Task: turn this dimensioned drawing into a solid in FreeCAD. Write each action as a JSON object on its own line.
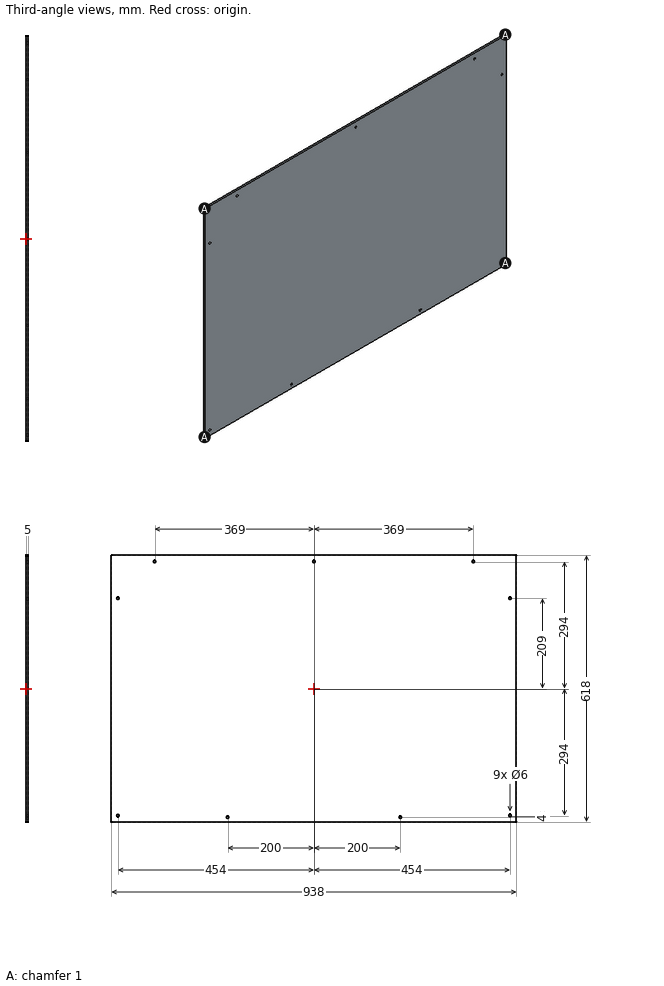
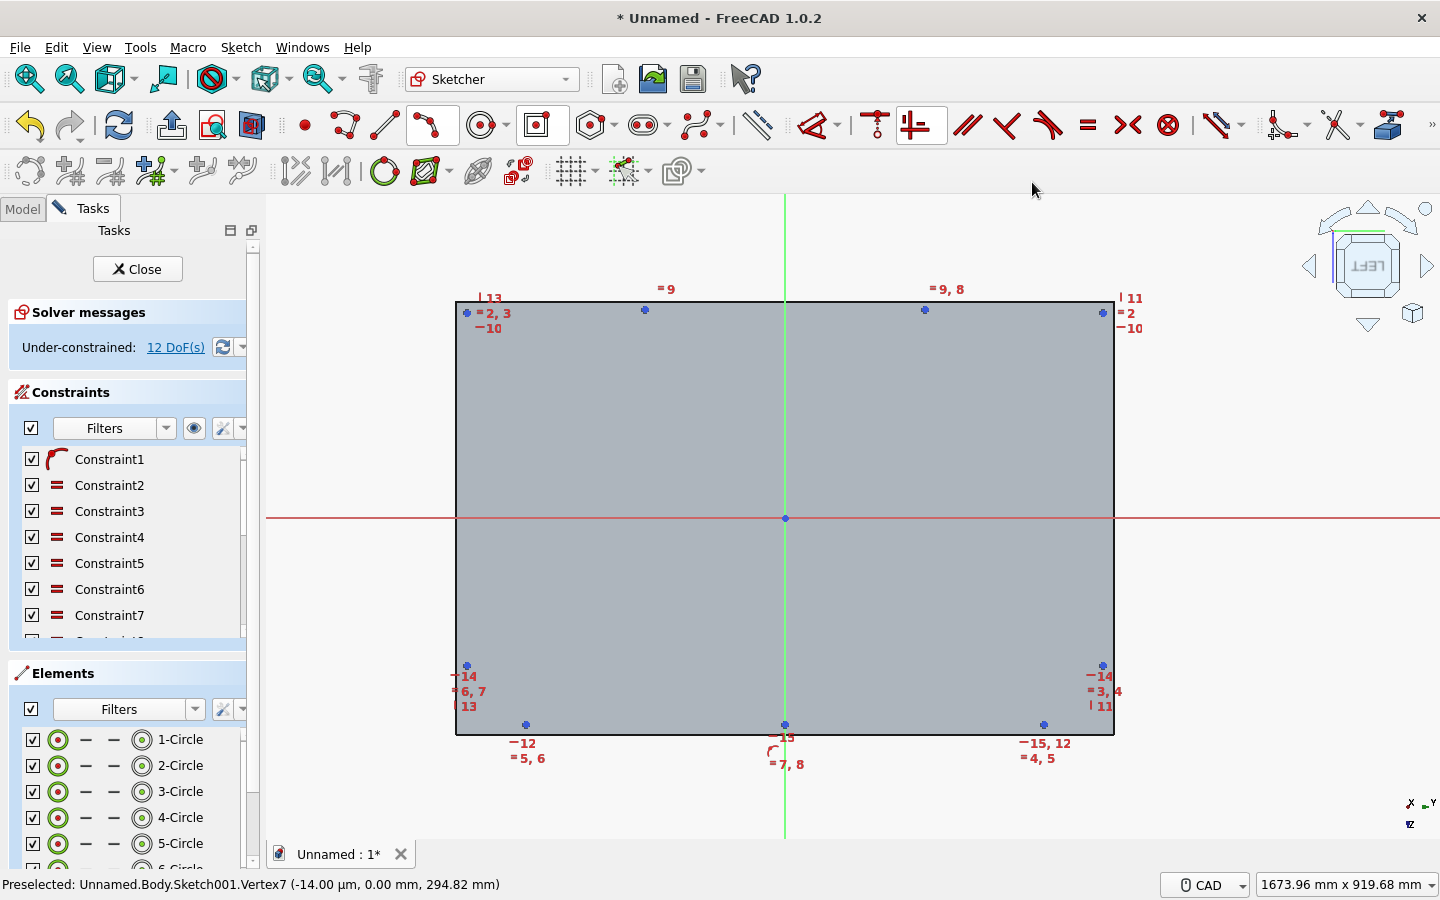
{"action": "left_click", "coordinate": [925, 310]}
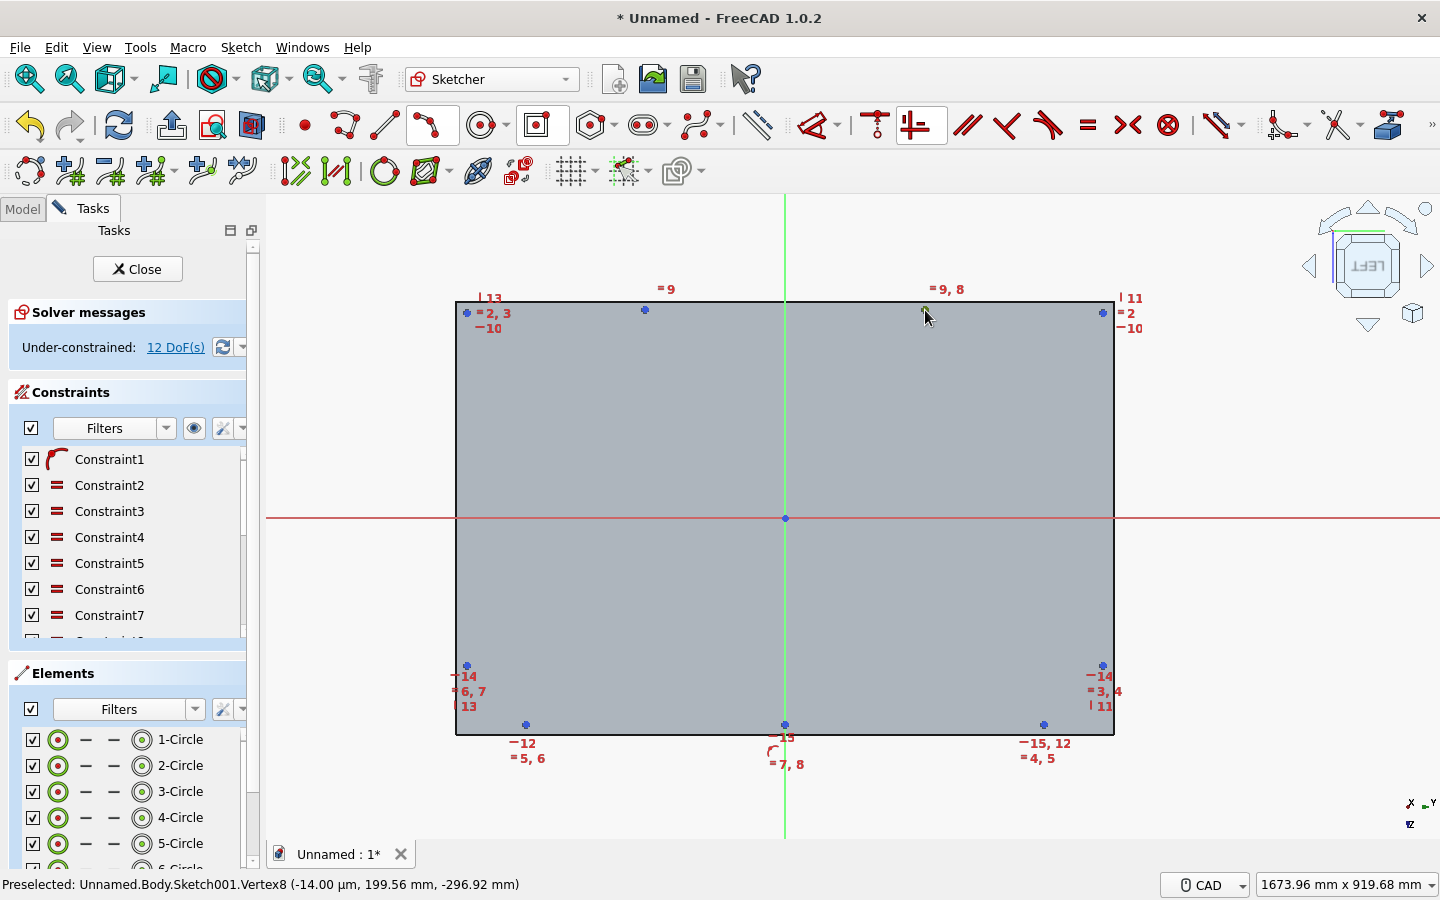
{"action": "left_click", "coordinate": [645, 310]}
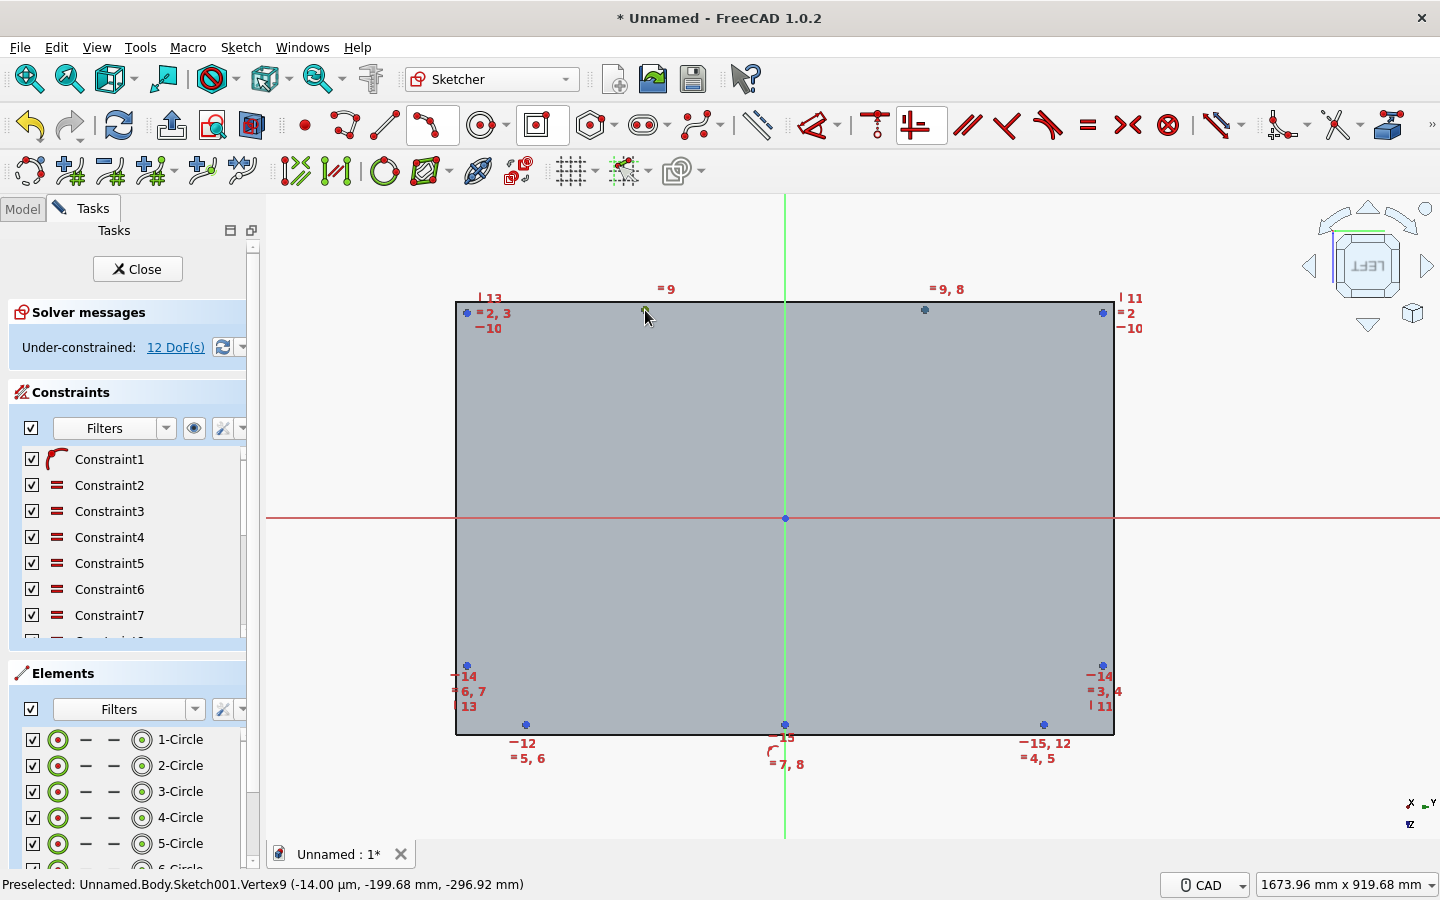
{"action": "key", "text": "h"}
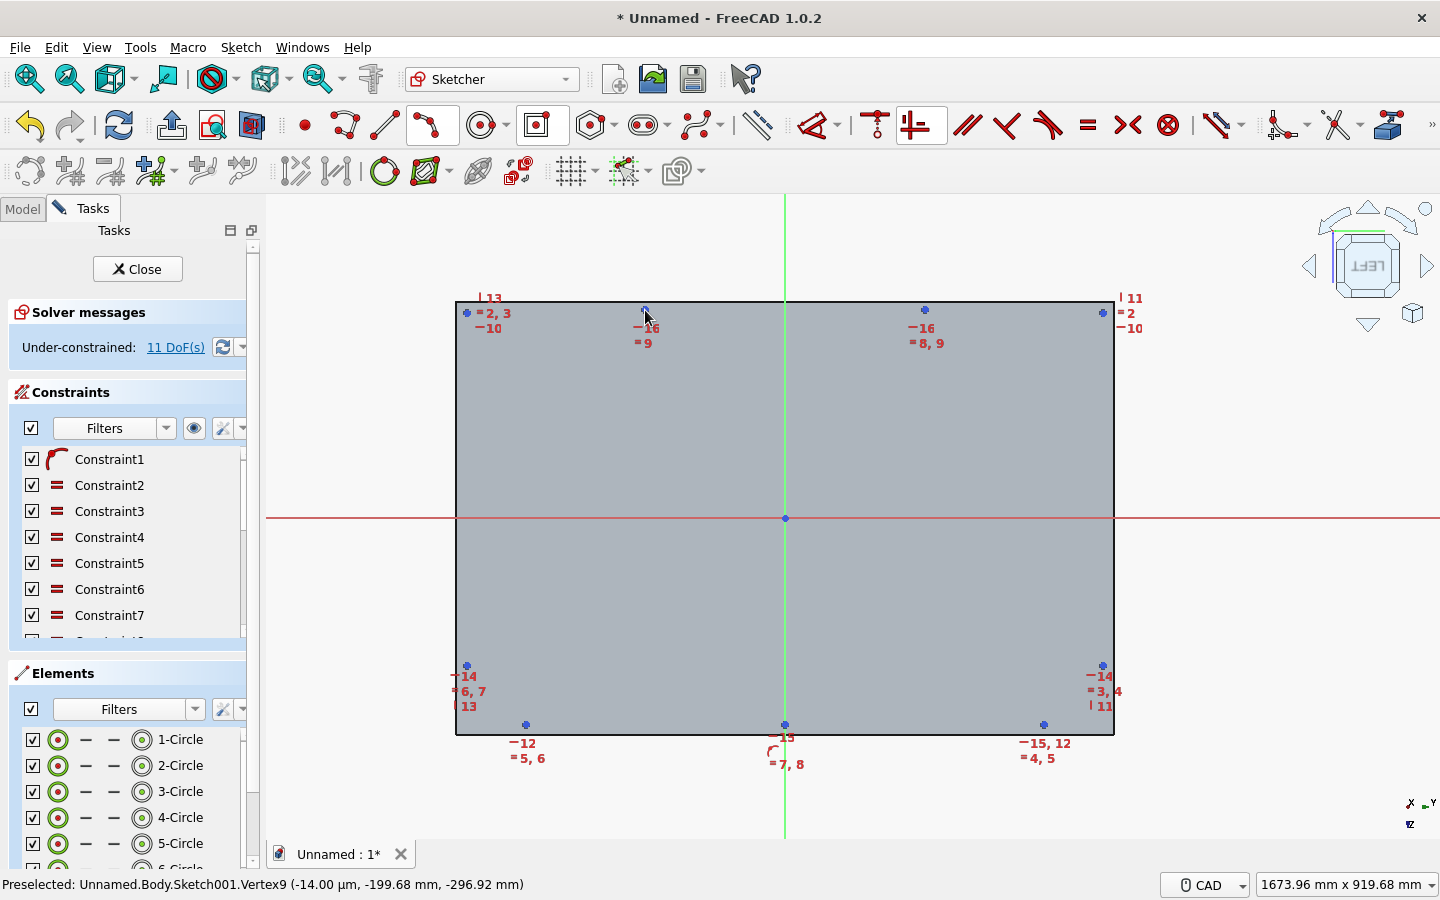
{"action": "left_click", "coordinate": [812, 126]}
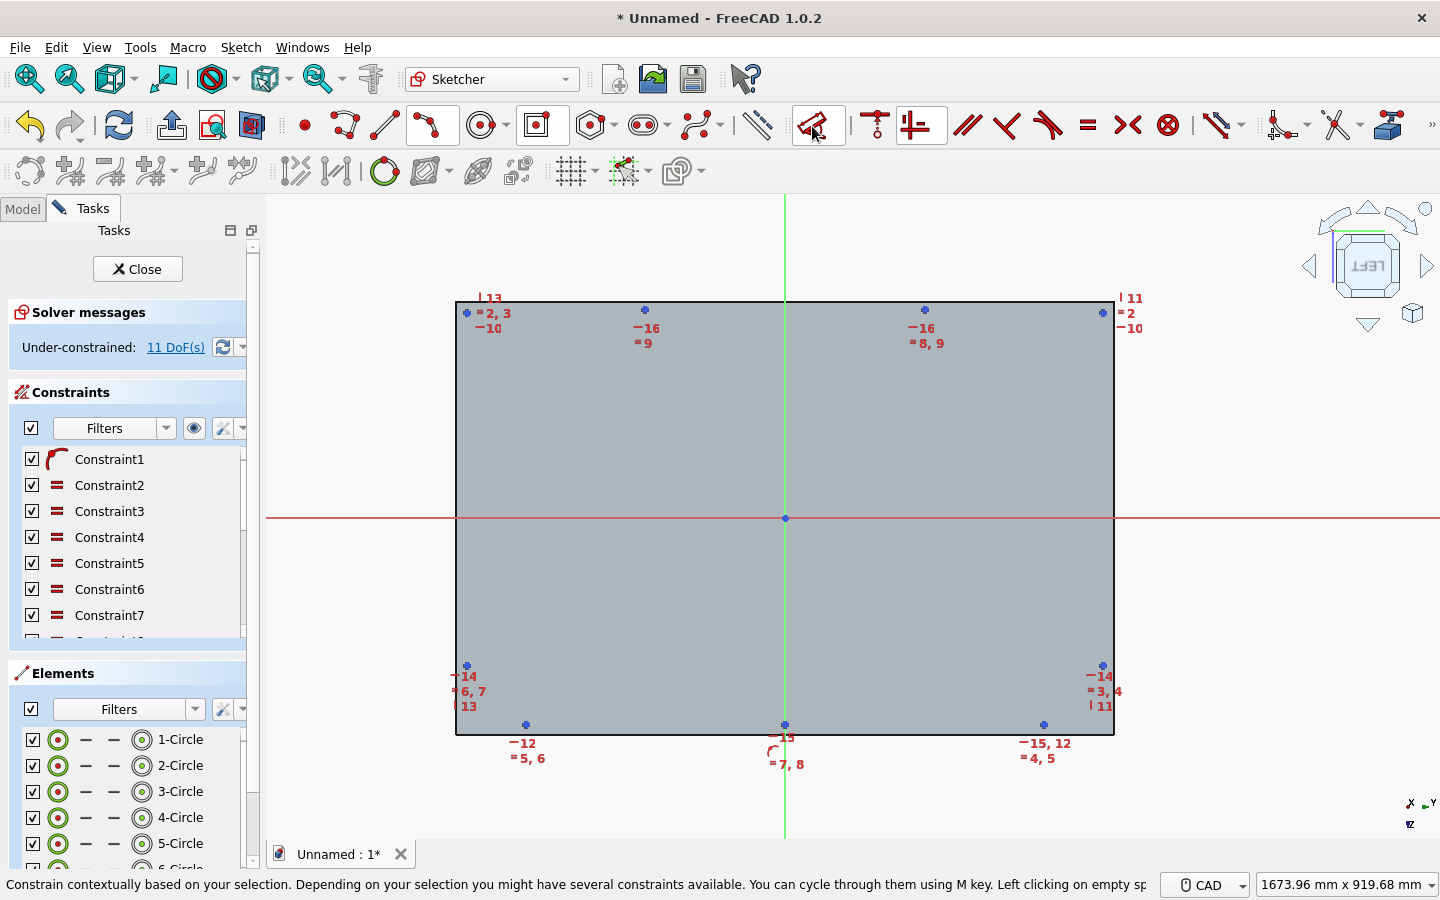
{"action": "scroll", "coordinate": [1105, 311], "scroll_direction": "up", "scroll_amount": 12}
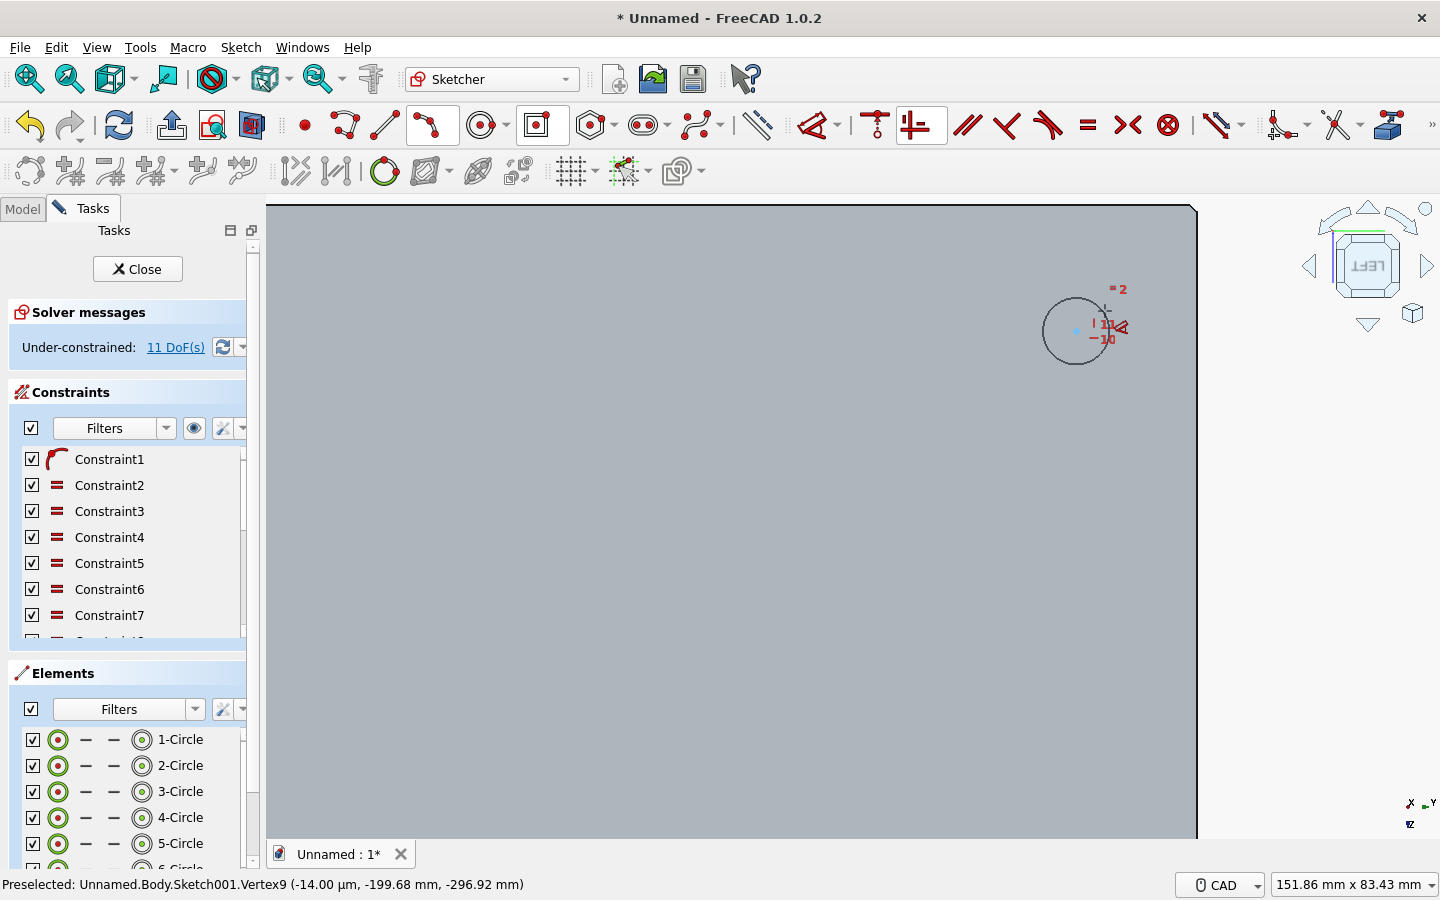
{"action": "left_click", "coordinate": [1100, 308]}
{"action": "left_click", "coordinate": [1123, 286]}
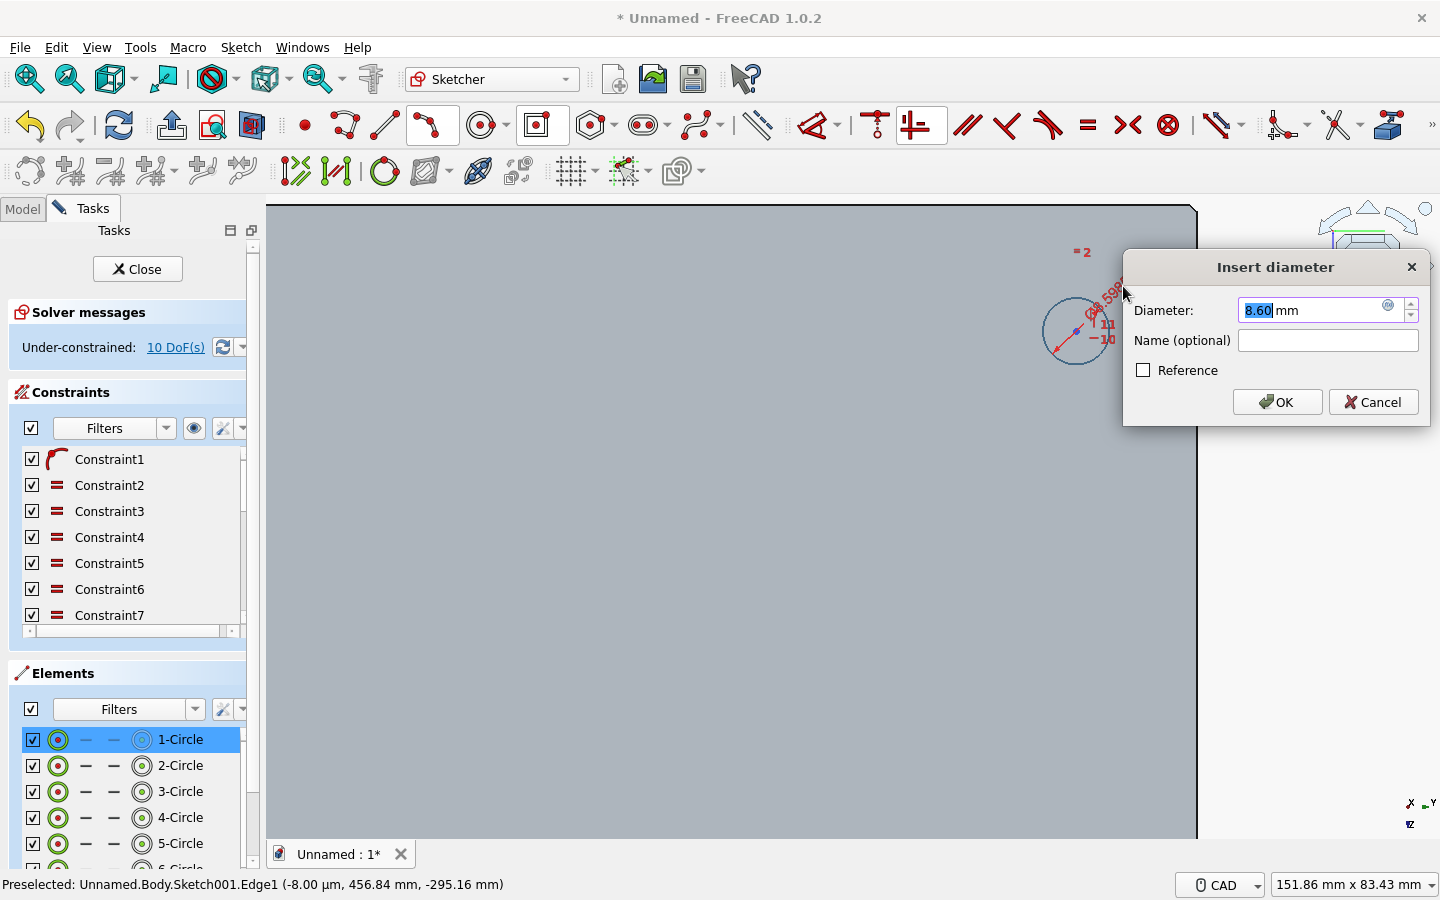
{"action": "type", "text": "6"}
{"action": "key", "text": "Return"}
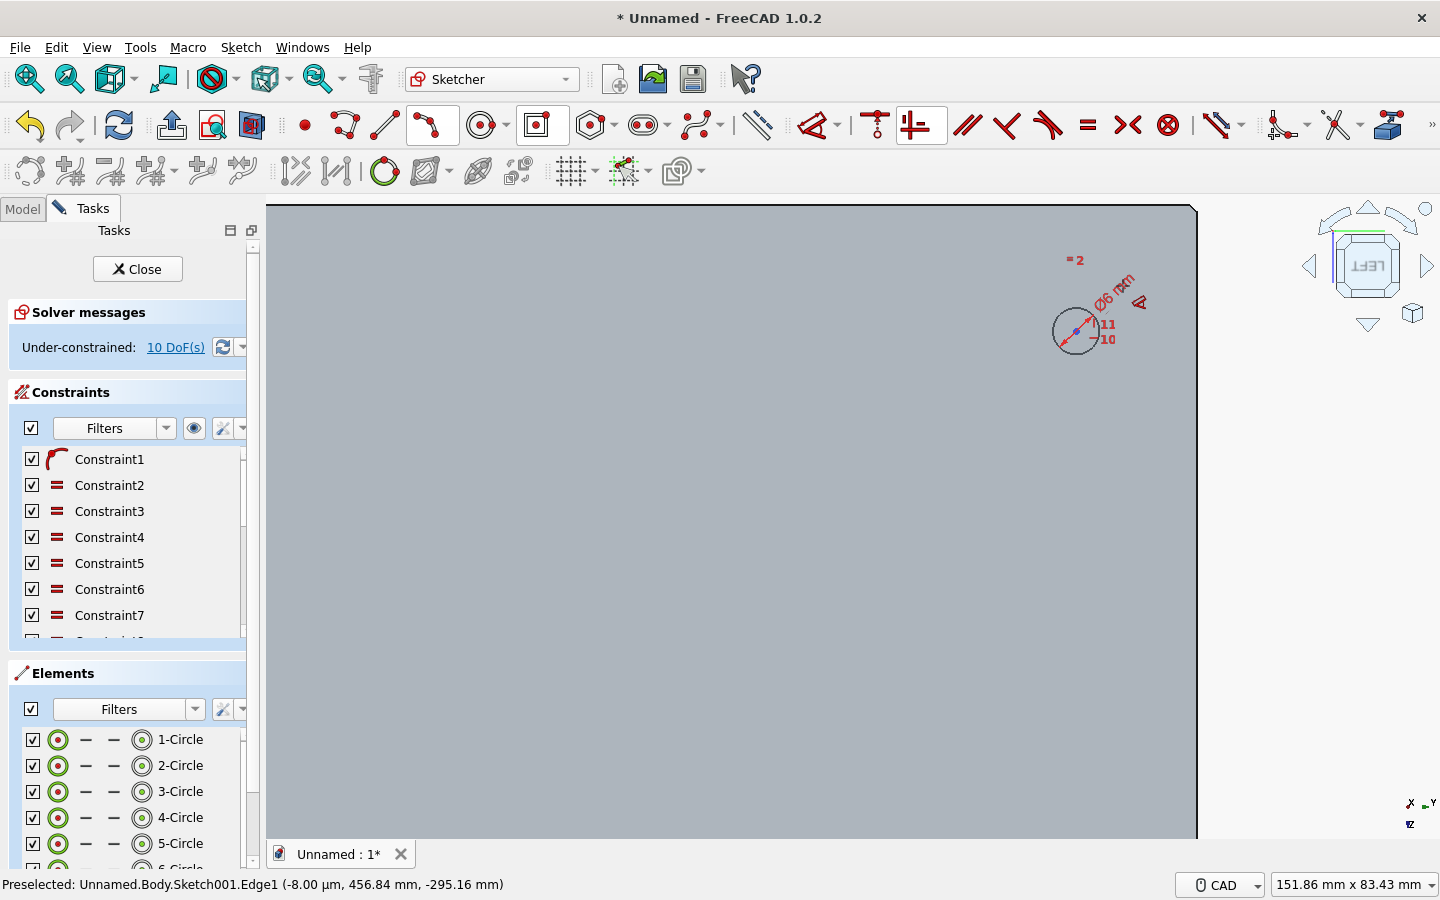
{"action": "scroll", "coordinate": [1076, 331], "scroll_direction": "up", "scroll_amount": 2}